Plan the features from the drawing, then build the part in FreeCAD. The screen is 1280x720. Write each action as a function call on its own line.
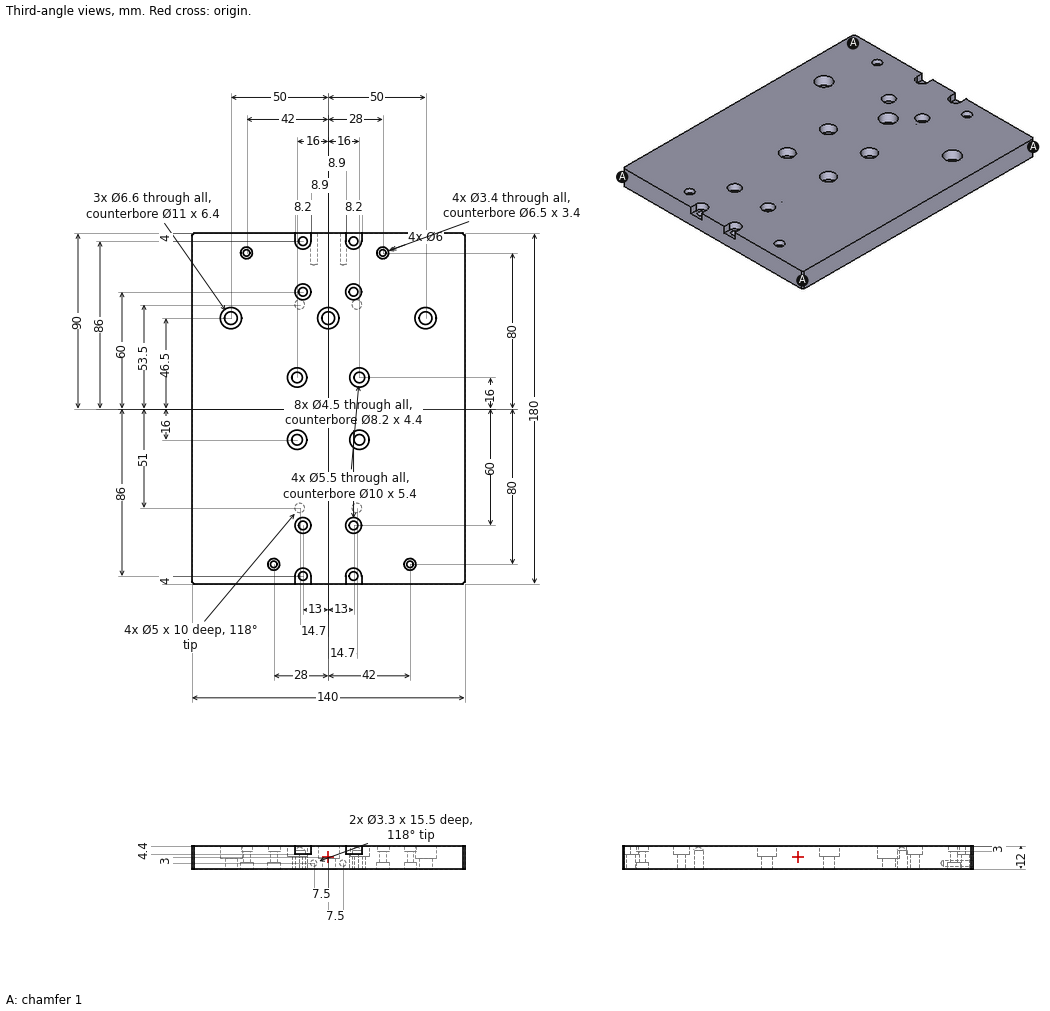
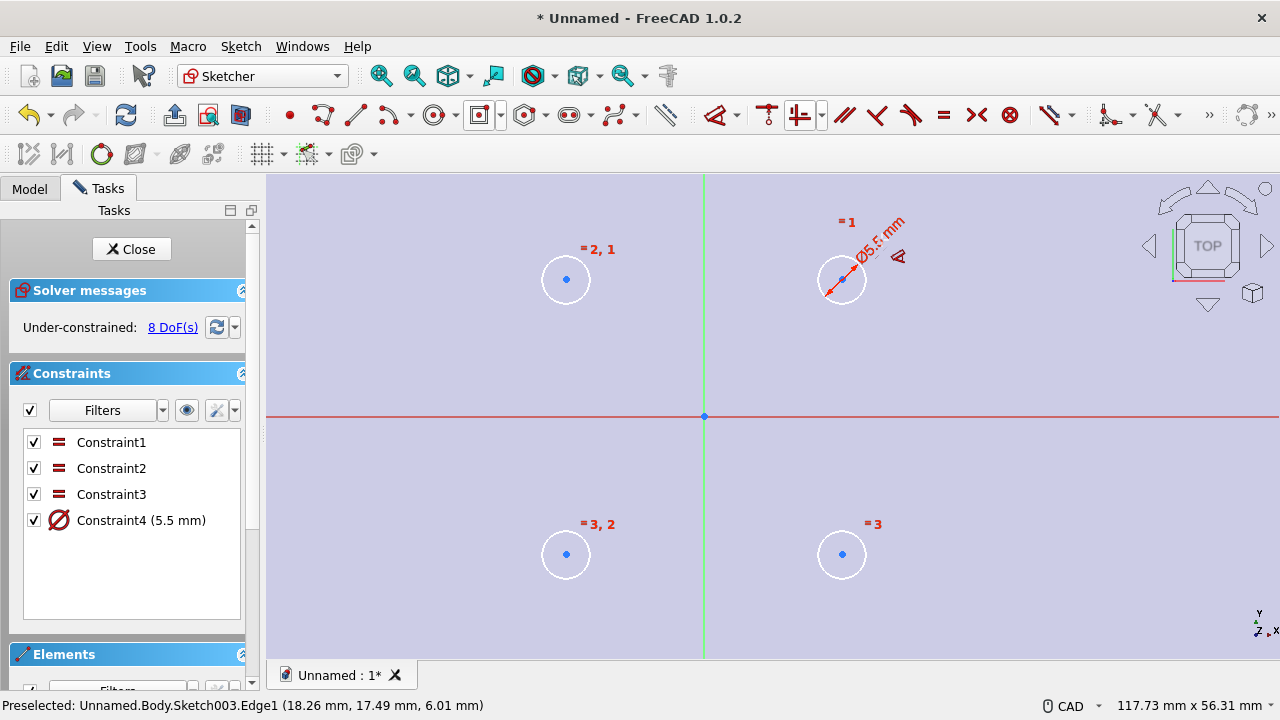
click(842, 280)
click(773, 246)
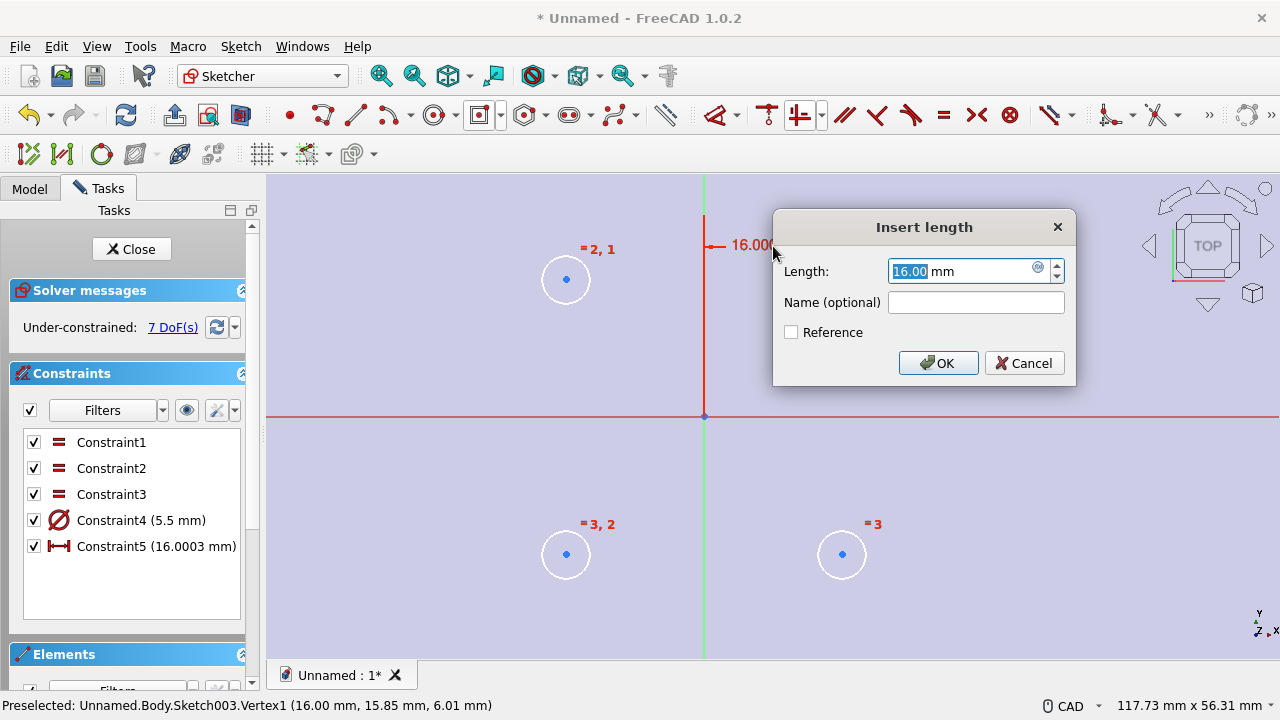
text(16)
key(Return)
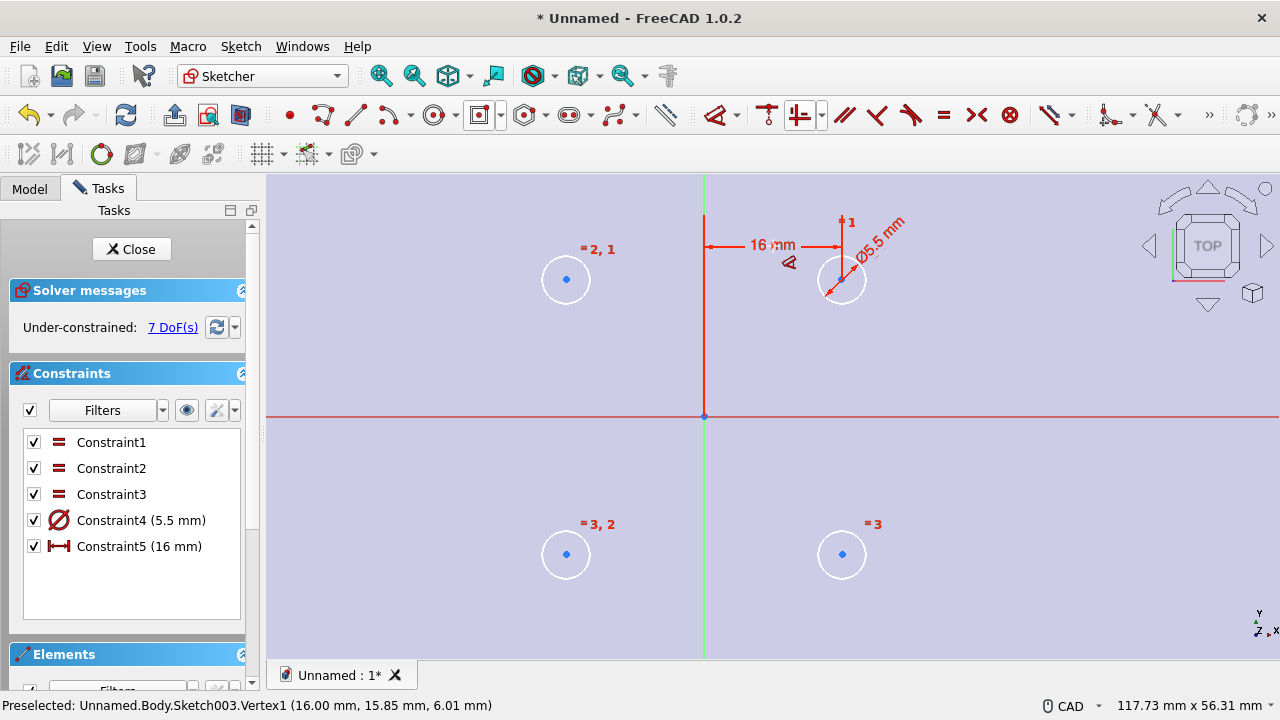
click(842, 280)
click(876, 348)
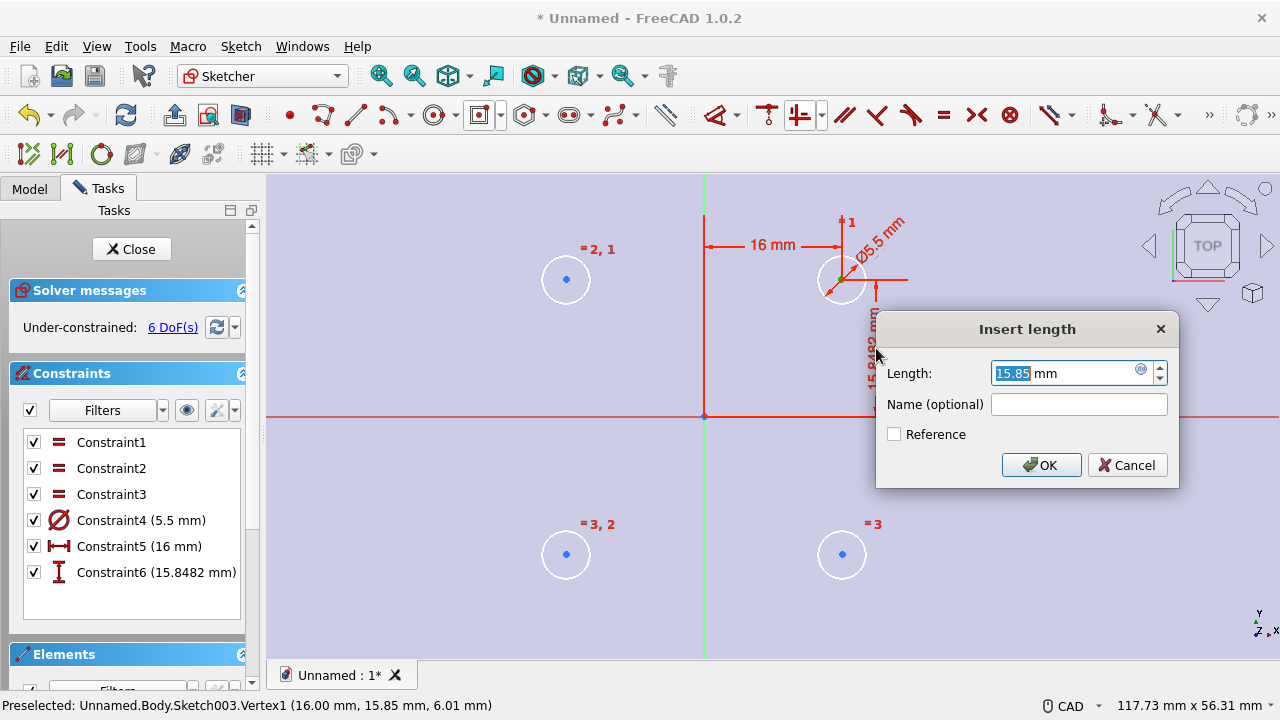
text(16)
key(Return)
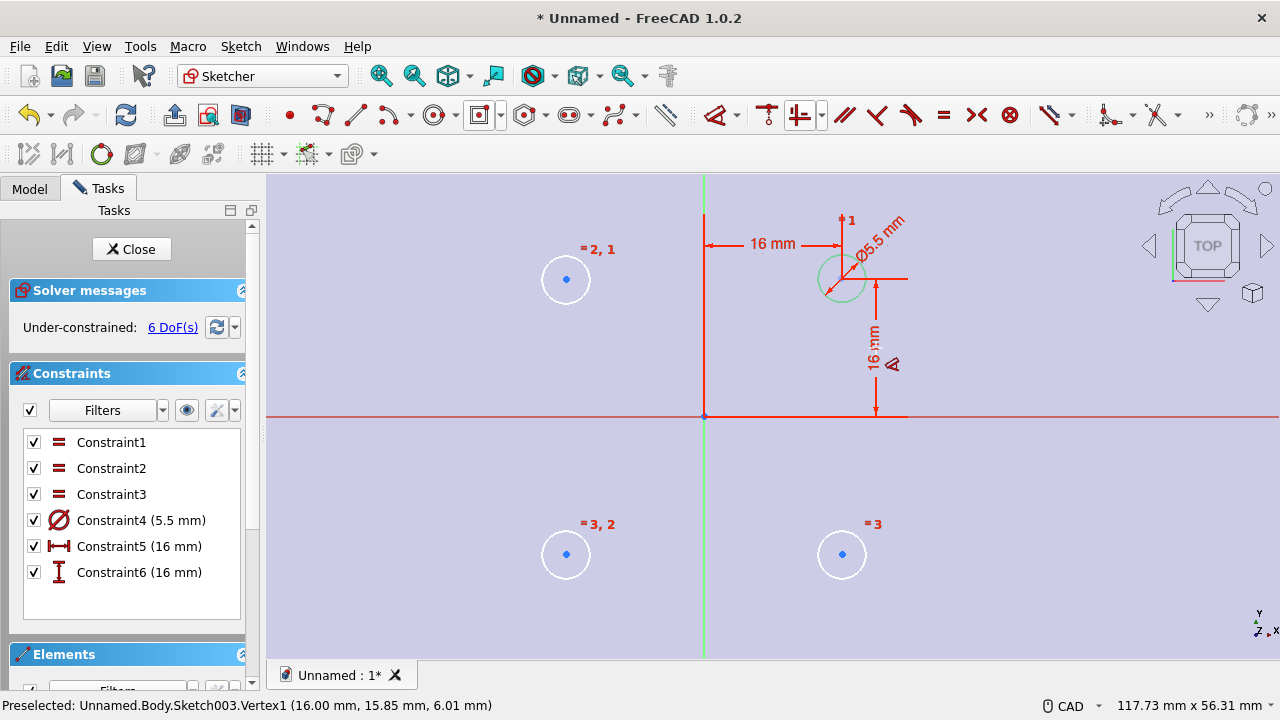
click(566, 280)
click(635, 246)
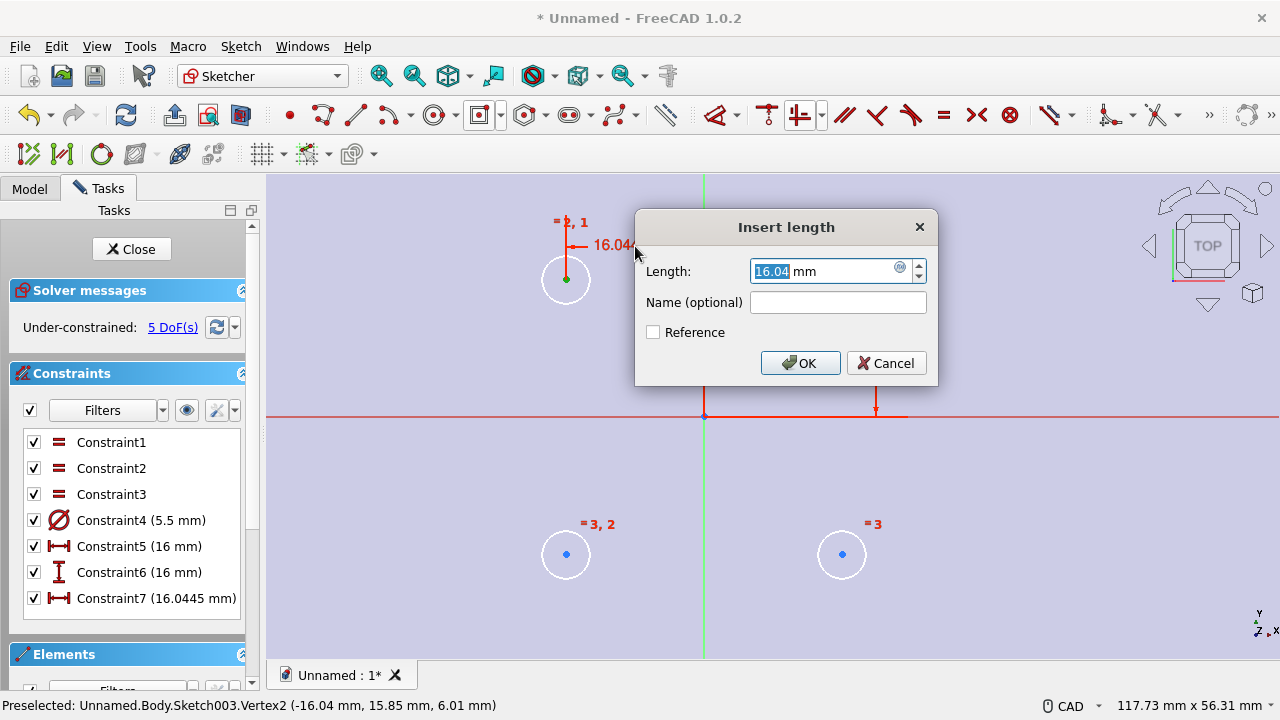
text(16)
key(Return)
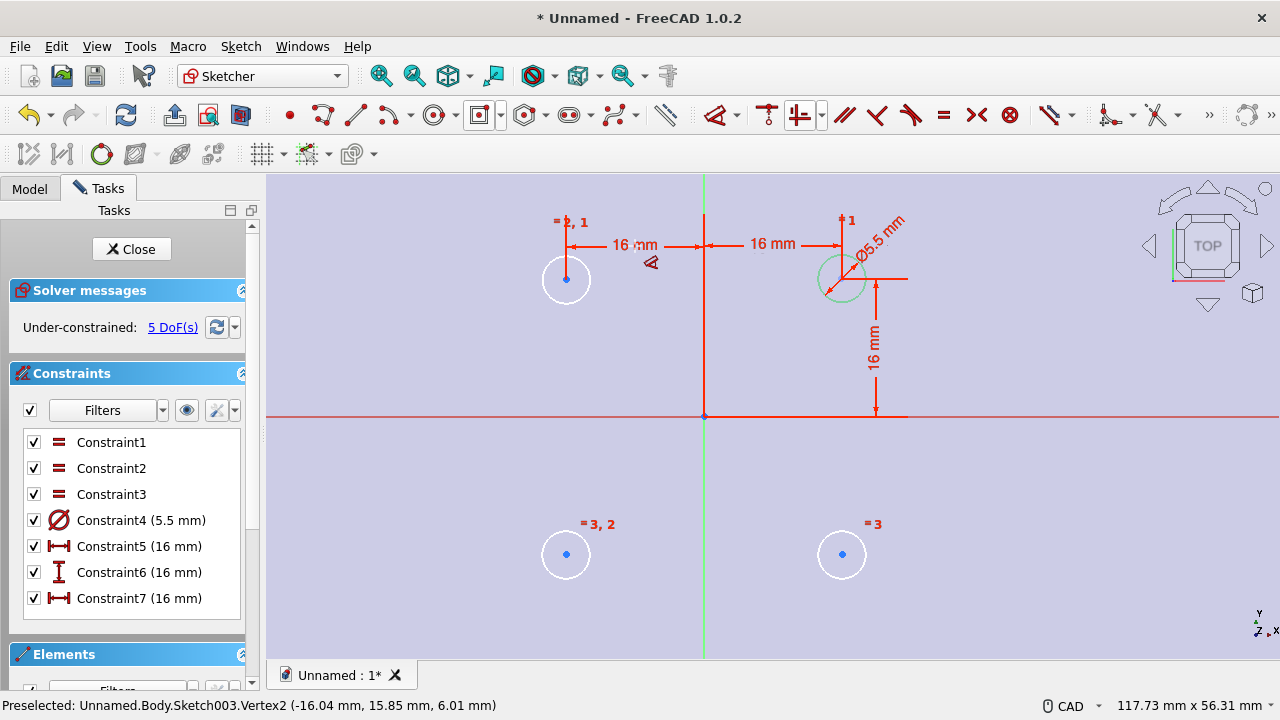
click(566, 280)
click(532, 348)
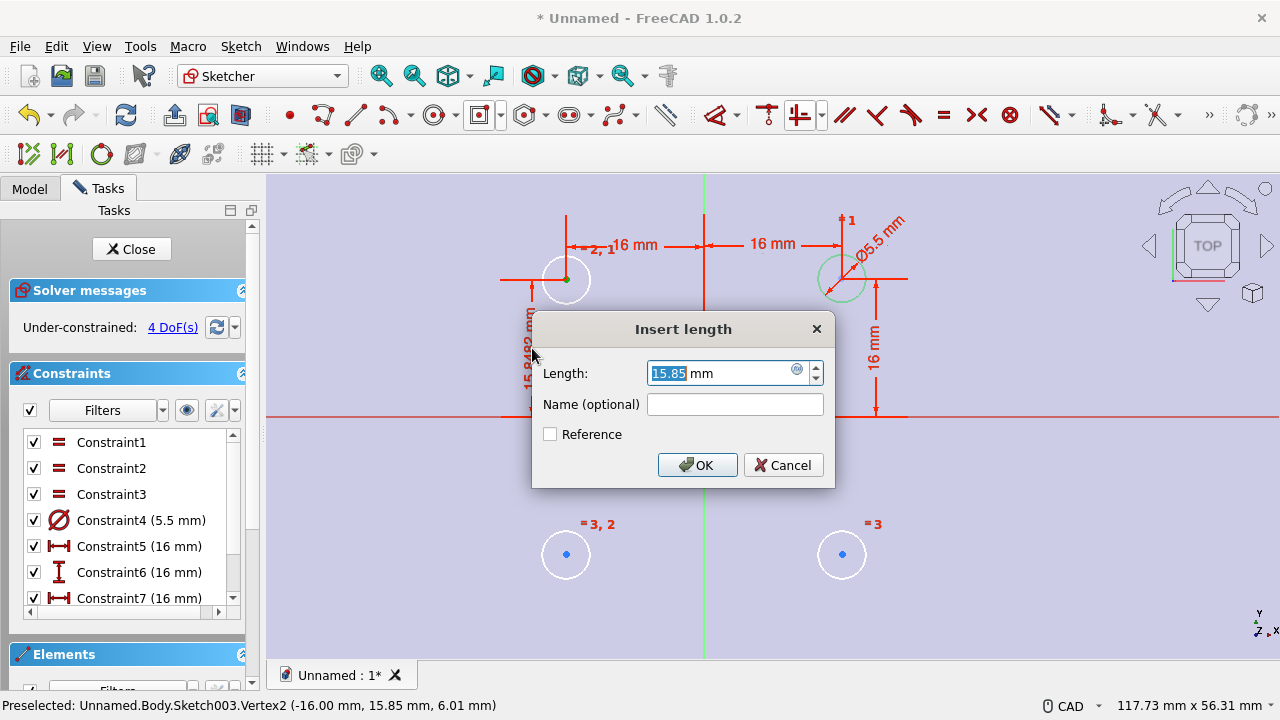
text(16)
key(Return)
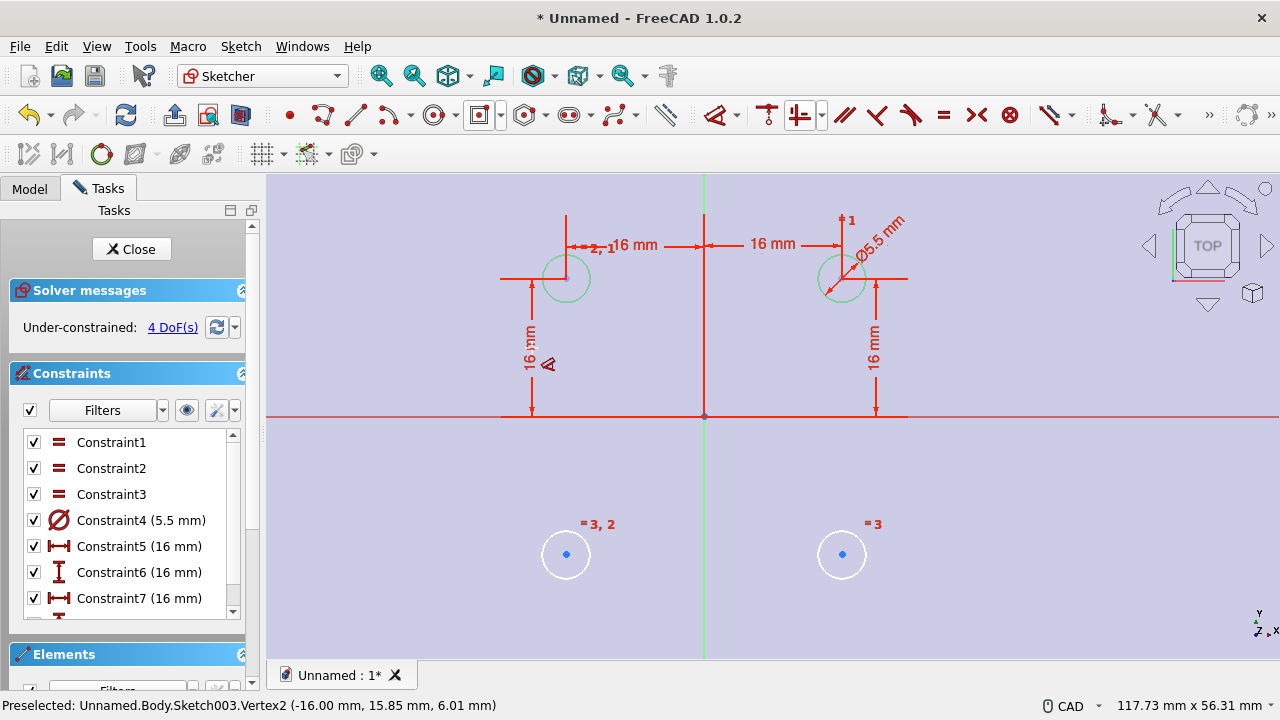
click(566, 555)
click(635, 589)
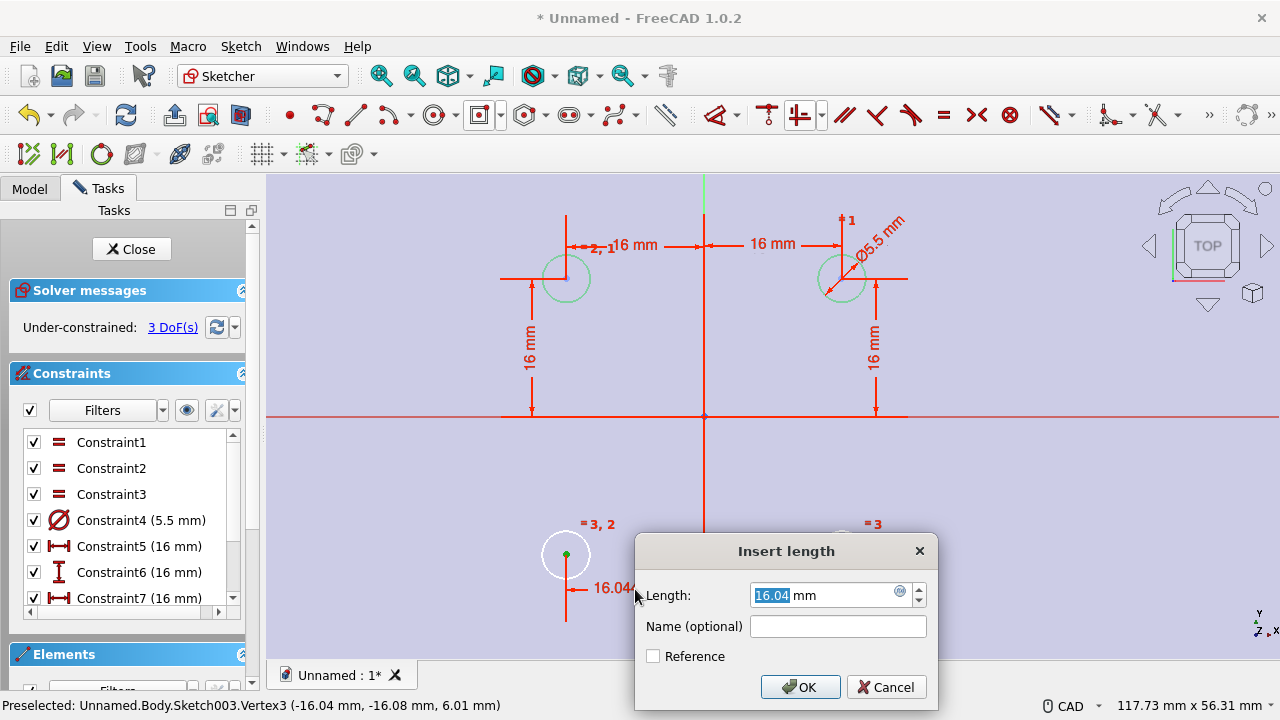
text(16)
key(Return)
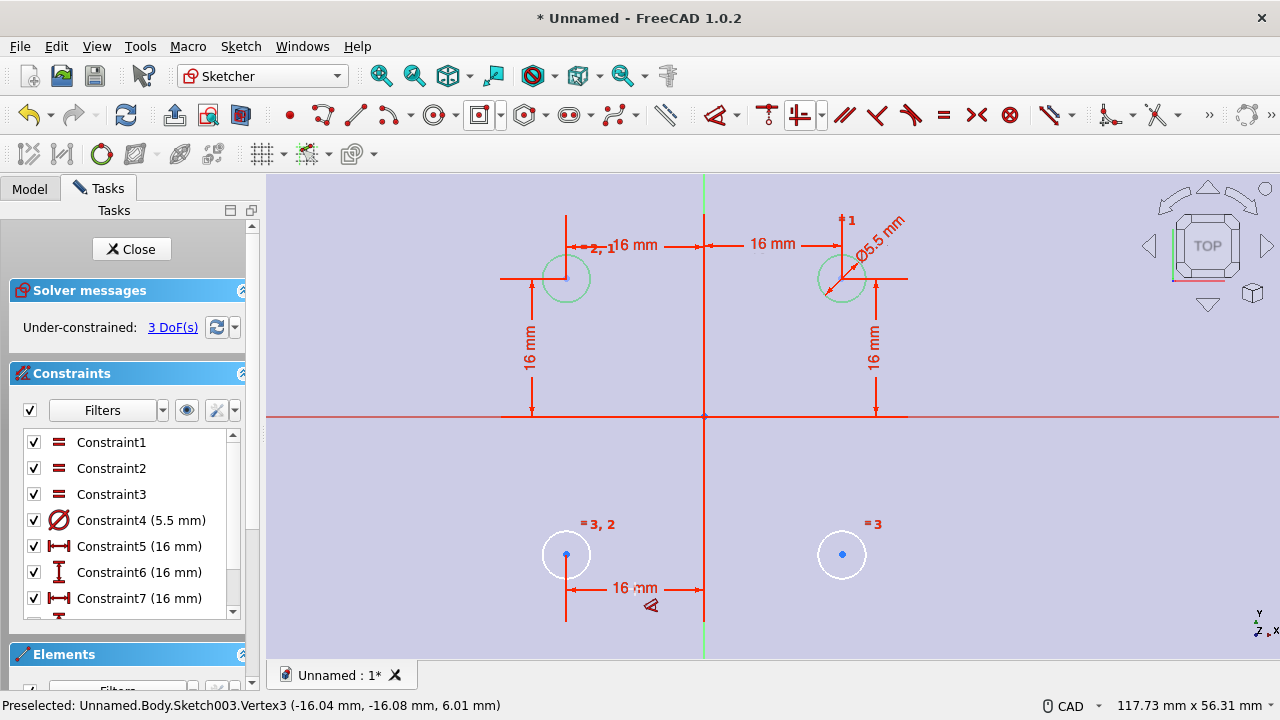
click(566, 555)
click(532, 486)